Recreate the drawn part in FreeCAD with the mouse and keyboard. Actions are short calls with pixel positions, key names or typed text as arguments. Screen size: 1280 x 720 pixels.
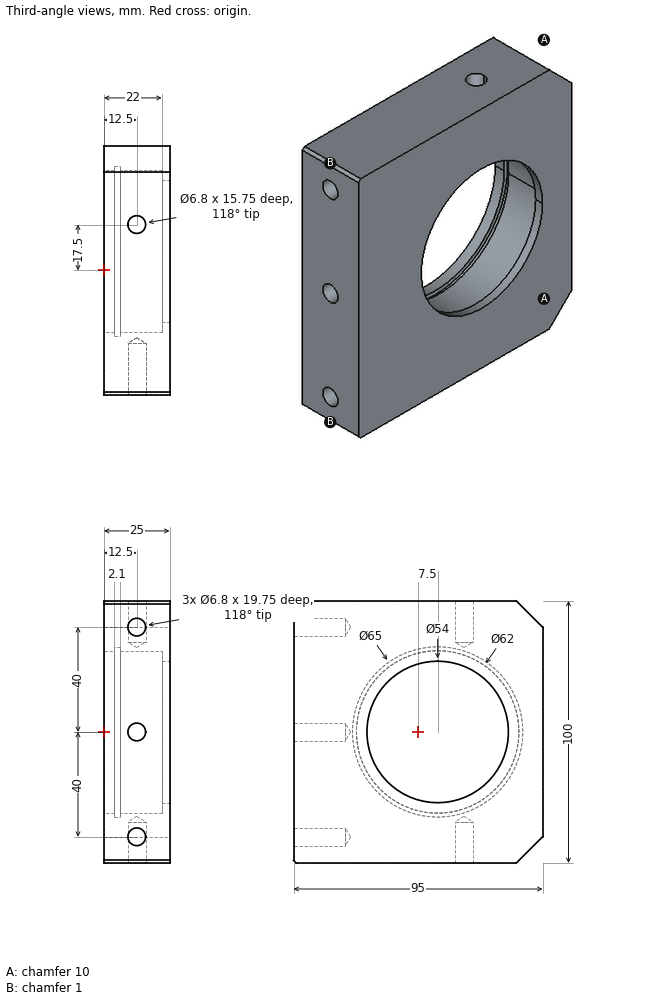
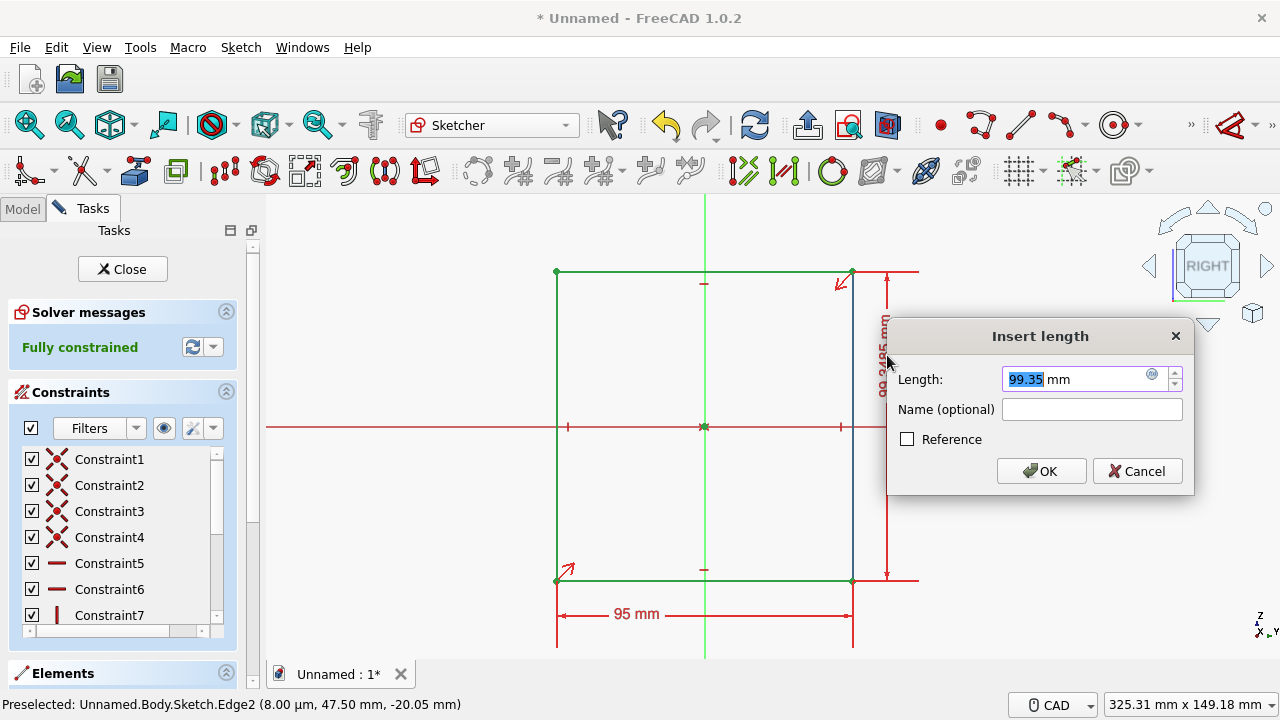
text(100)
key(Return)
key(Escape)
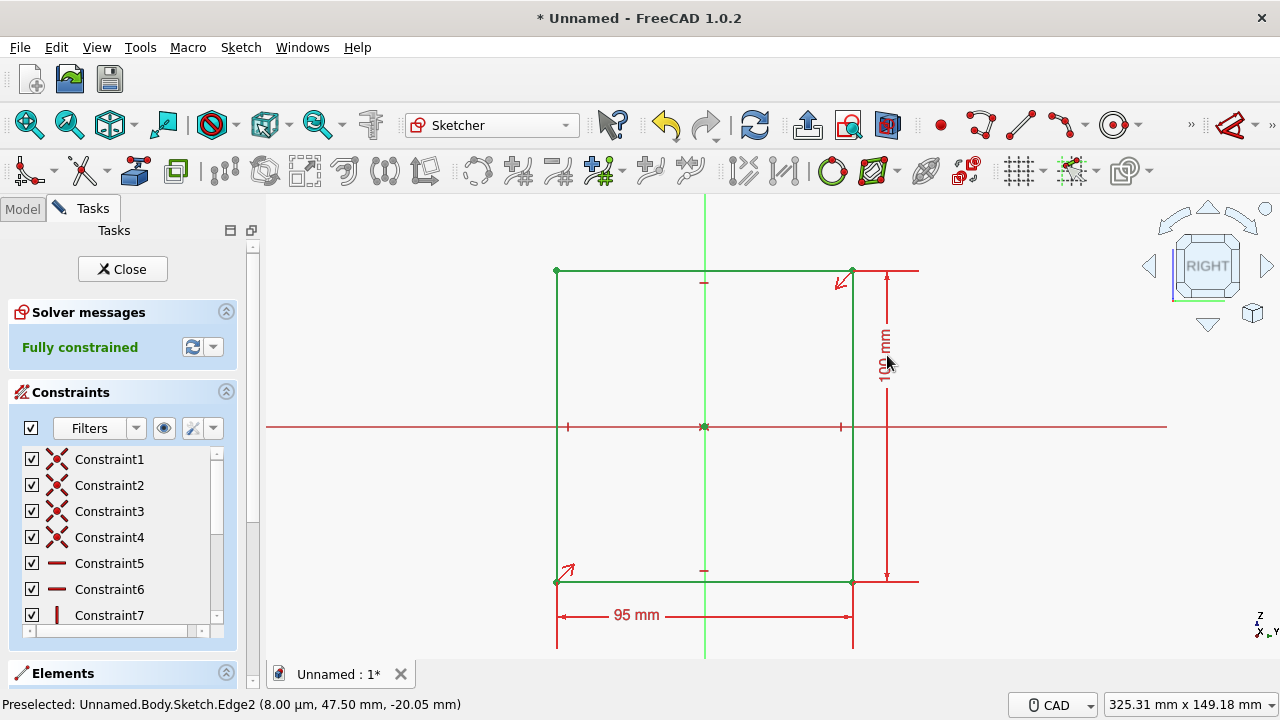
click(123, 269)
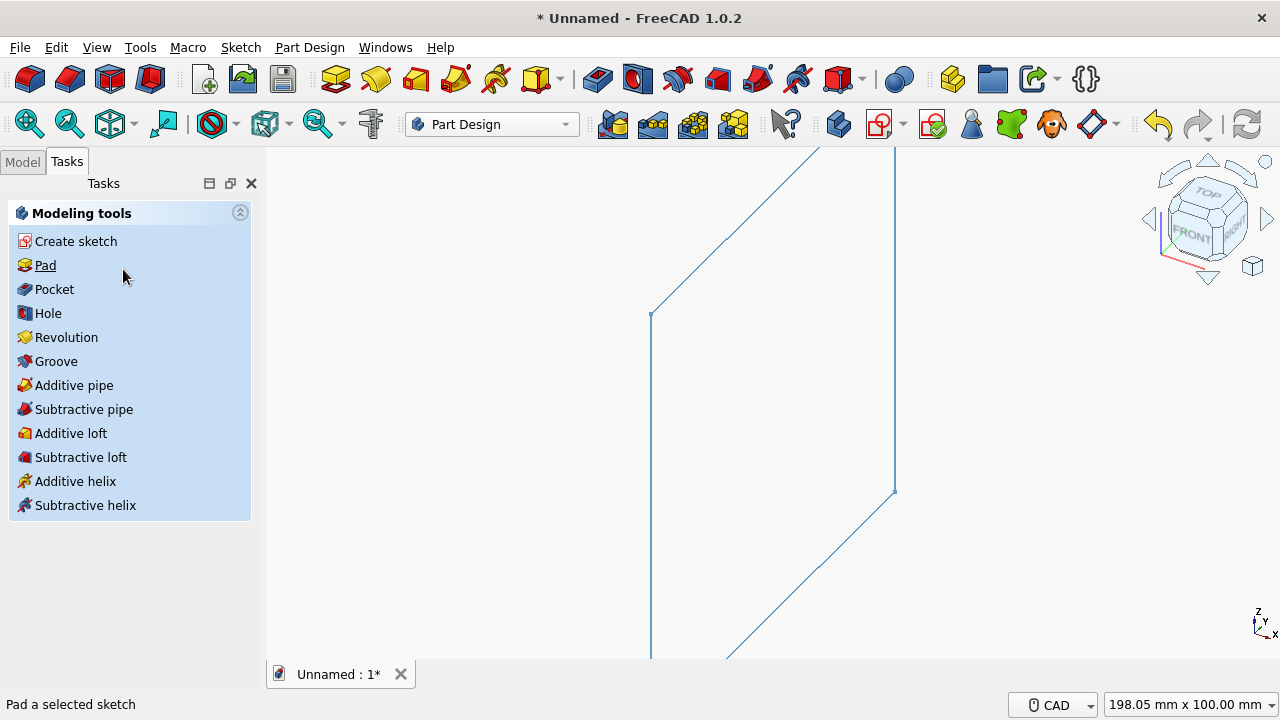
click(336, 80)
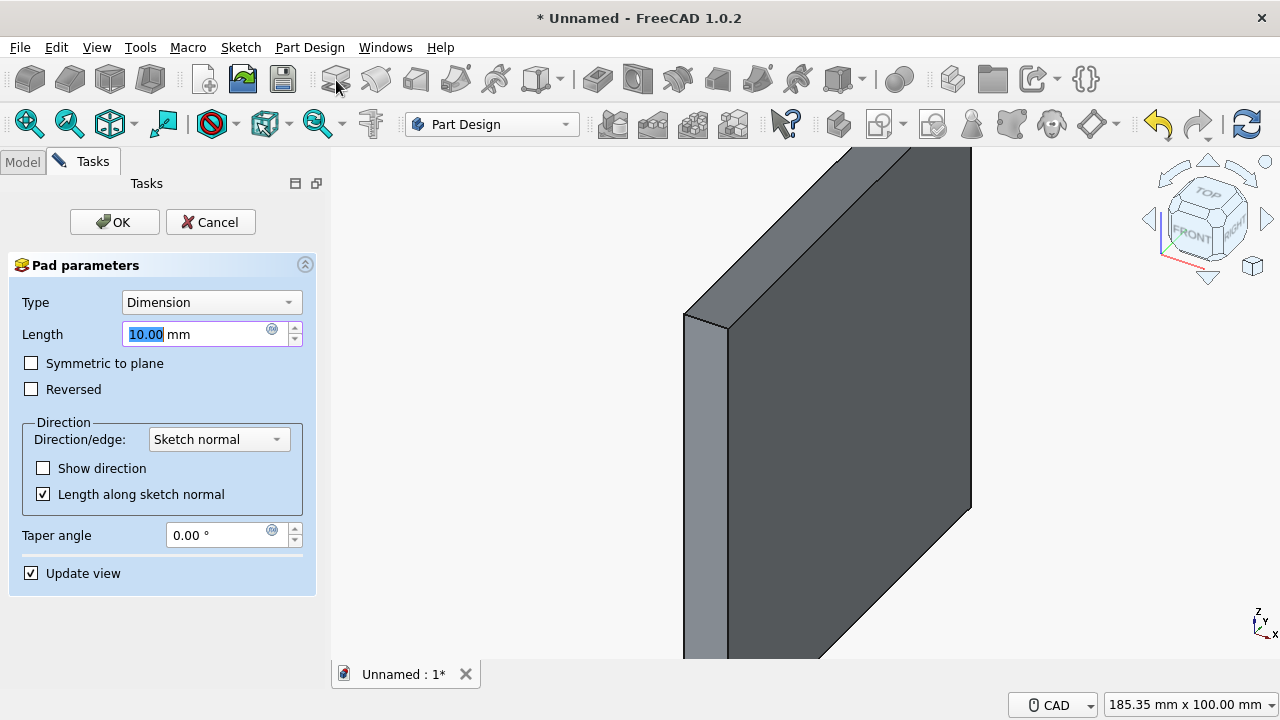
text(25)
key(Tab)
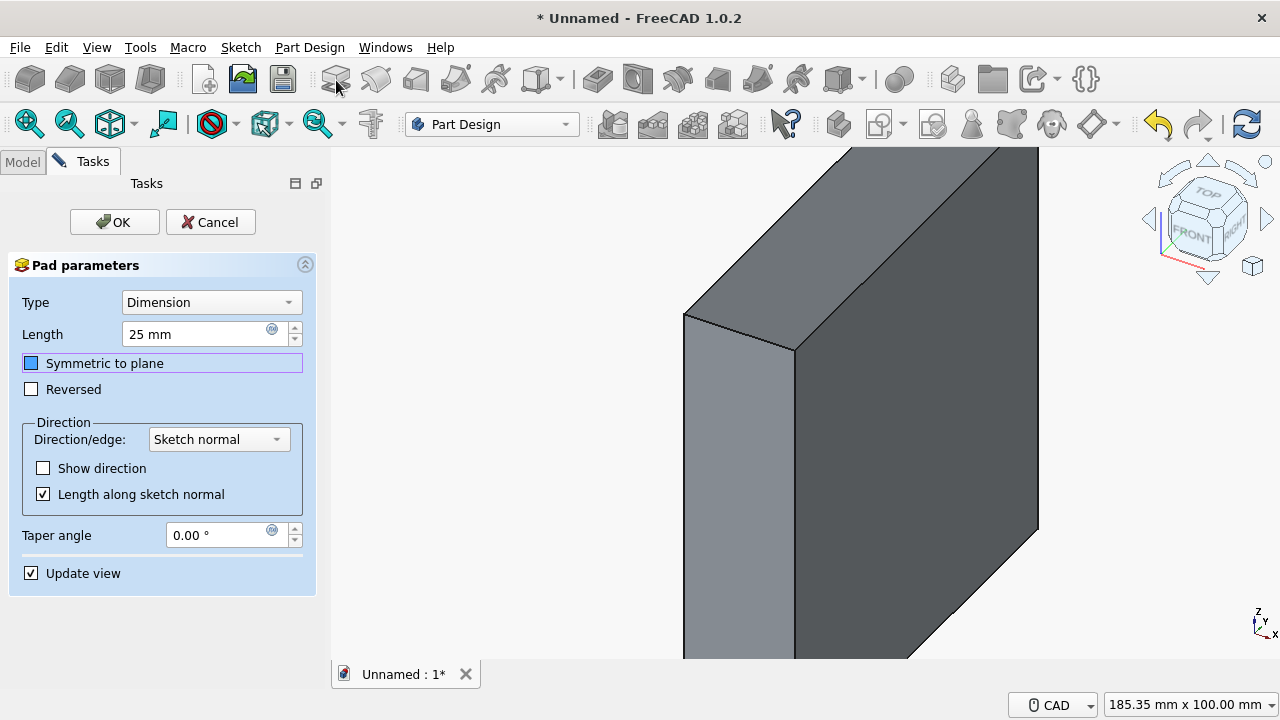
click(115, 222)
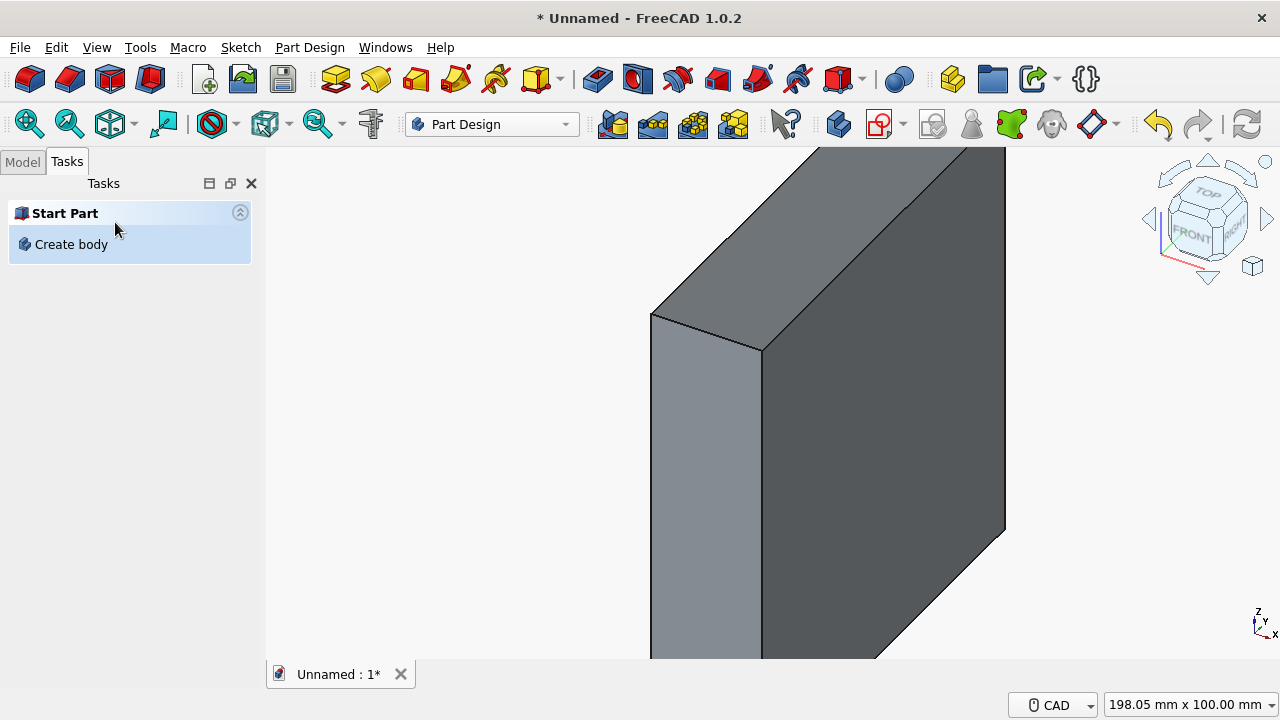
click(30, 124)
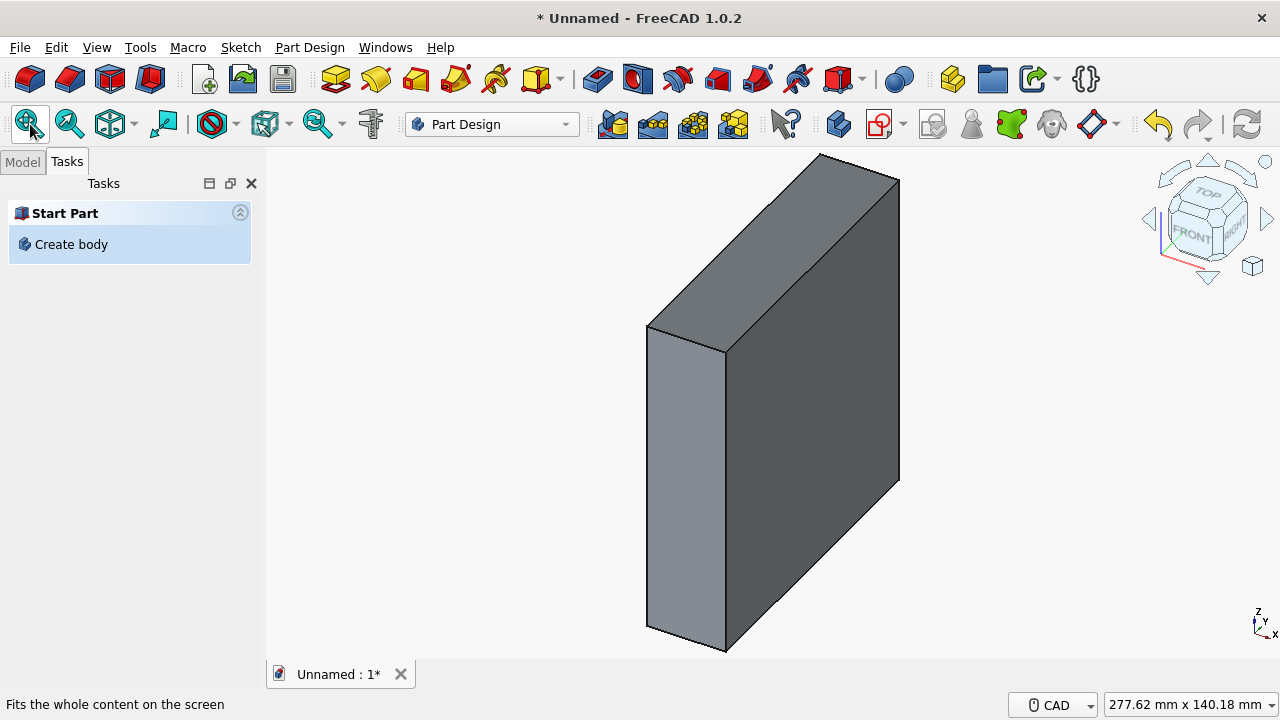
key(6)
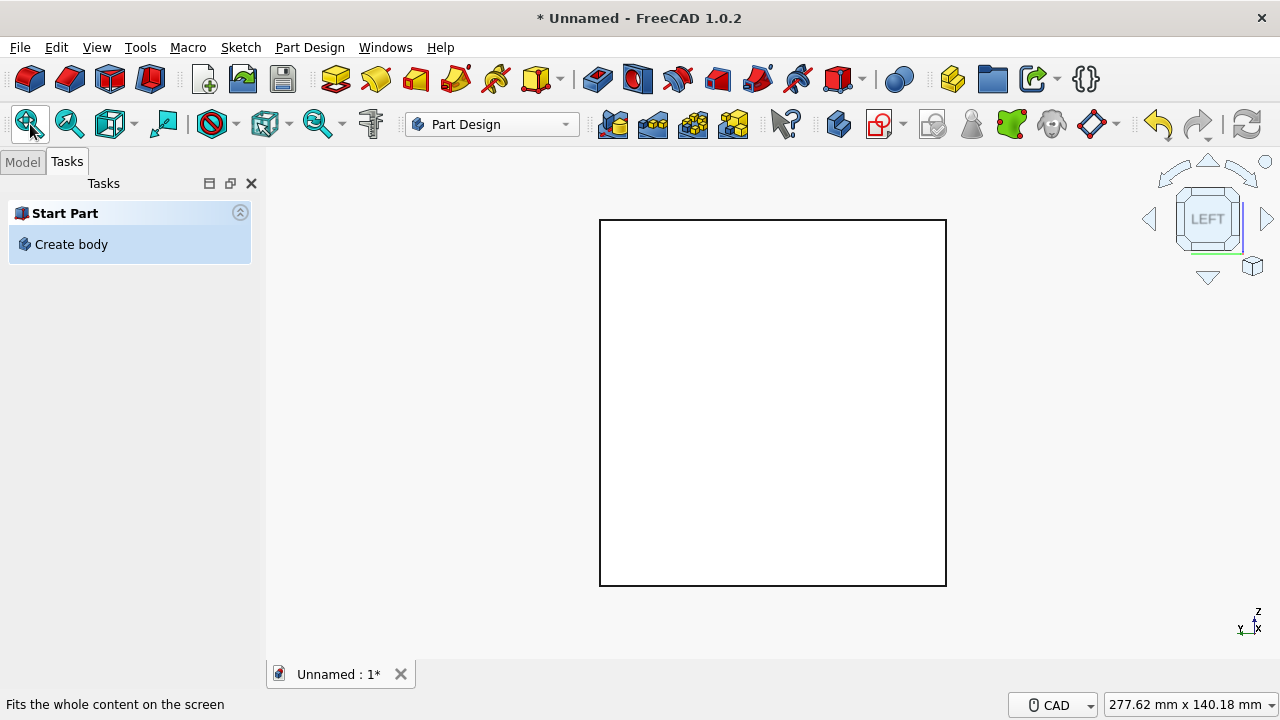
click(773, 402)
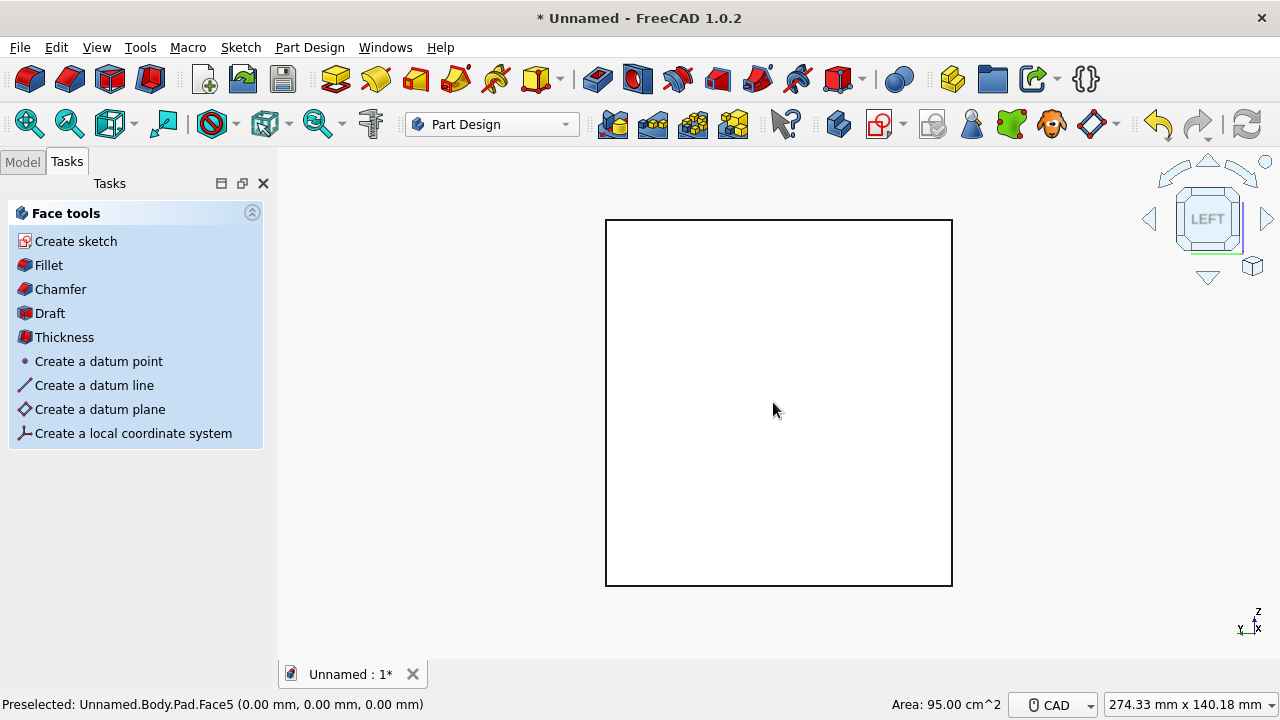
click(880, 124)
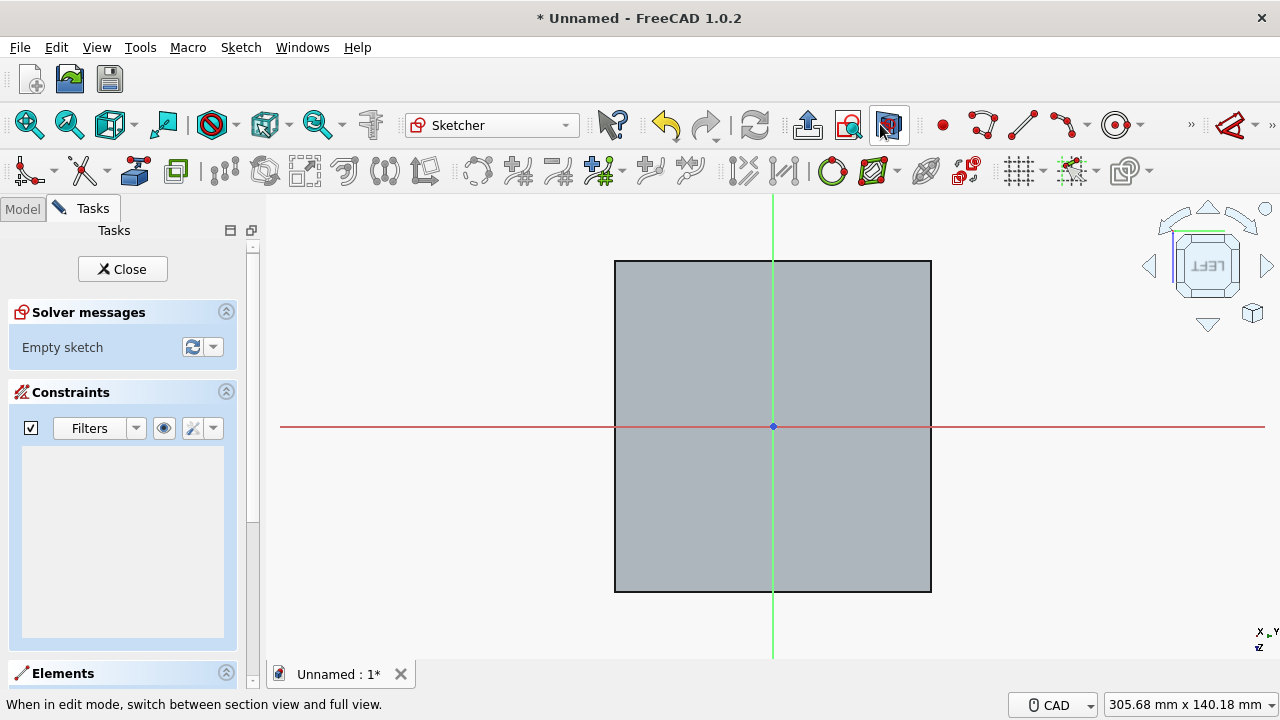
scroll(988, 426, up, 2)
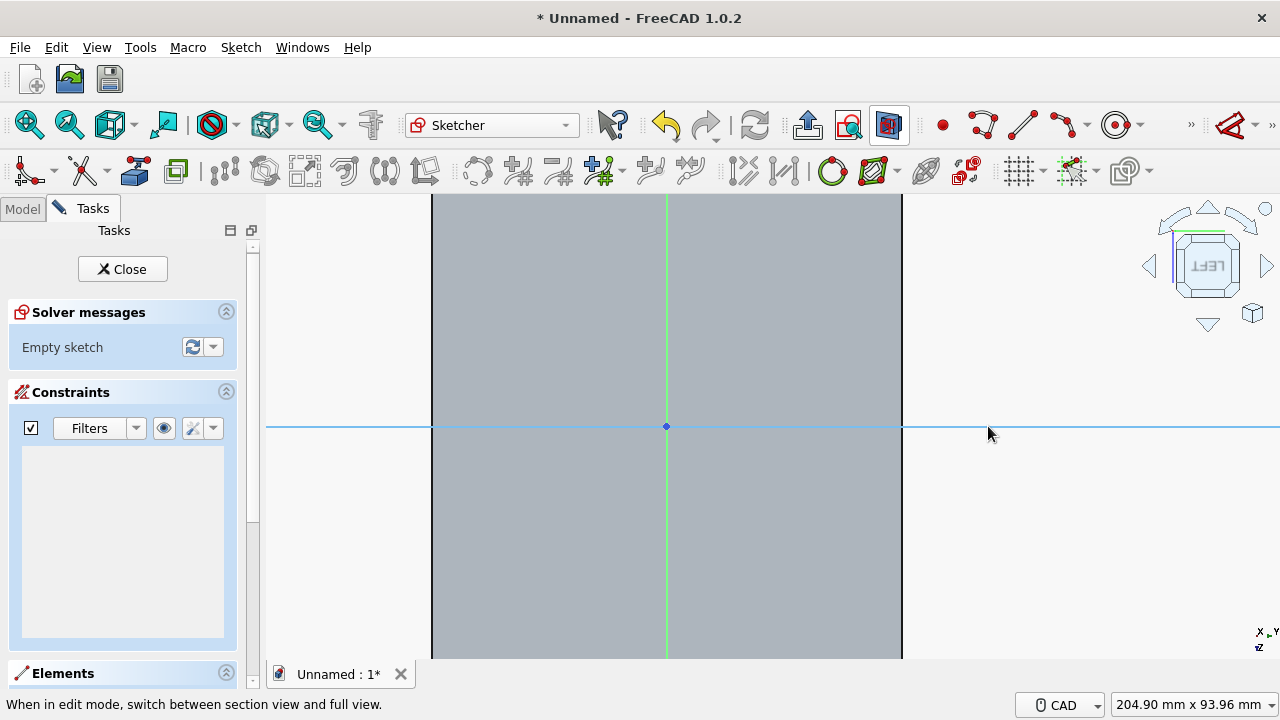
click(1116, 126)